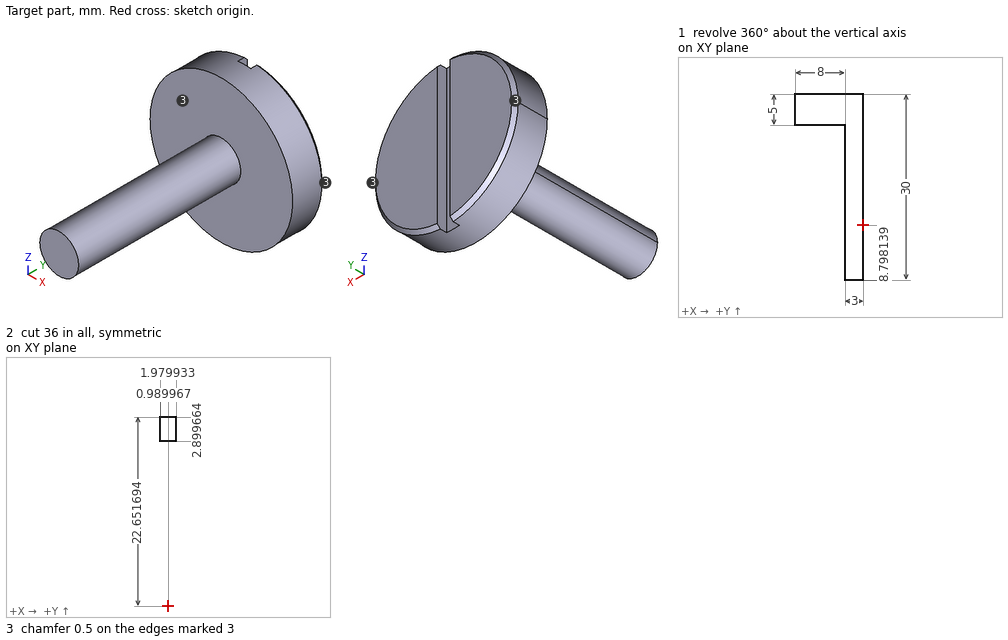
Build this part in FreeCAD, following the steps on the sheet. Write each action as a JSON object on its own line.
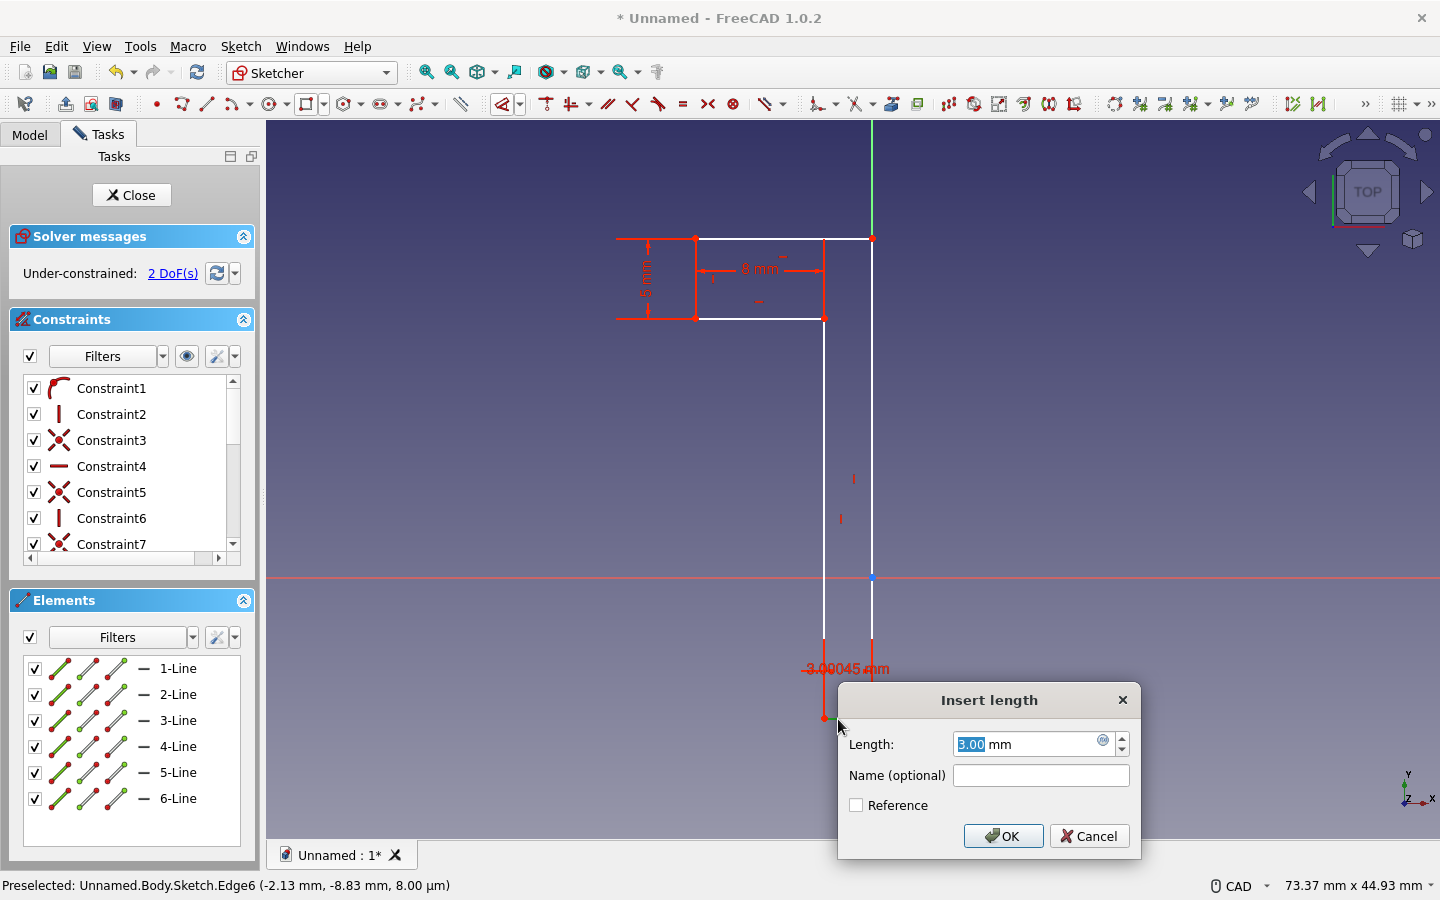
{"action": "type", "text": "3"}
{"action": "key", "text": "Return"}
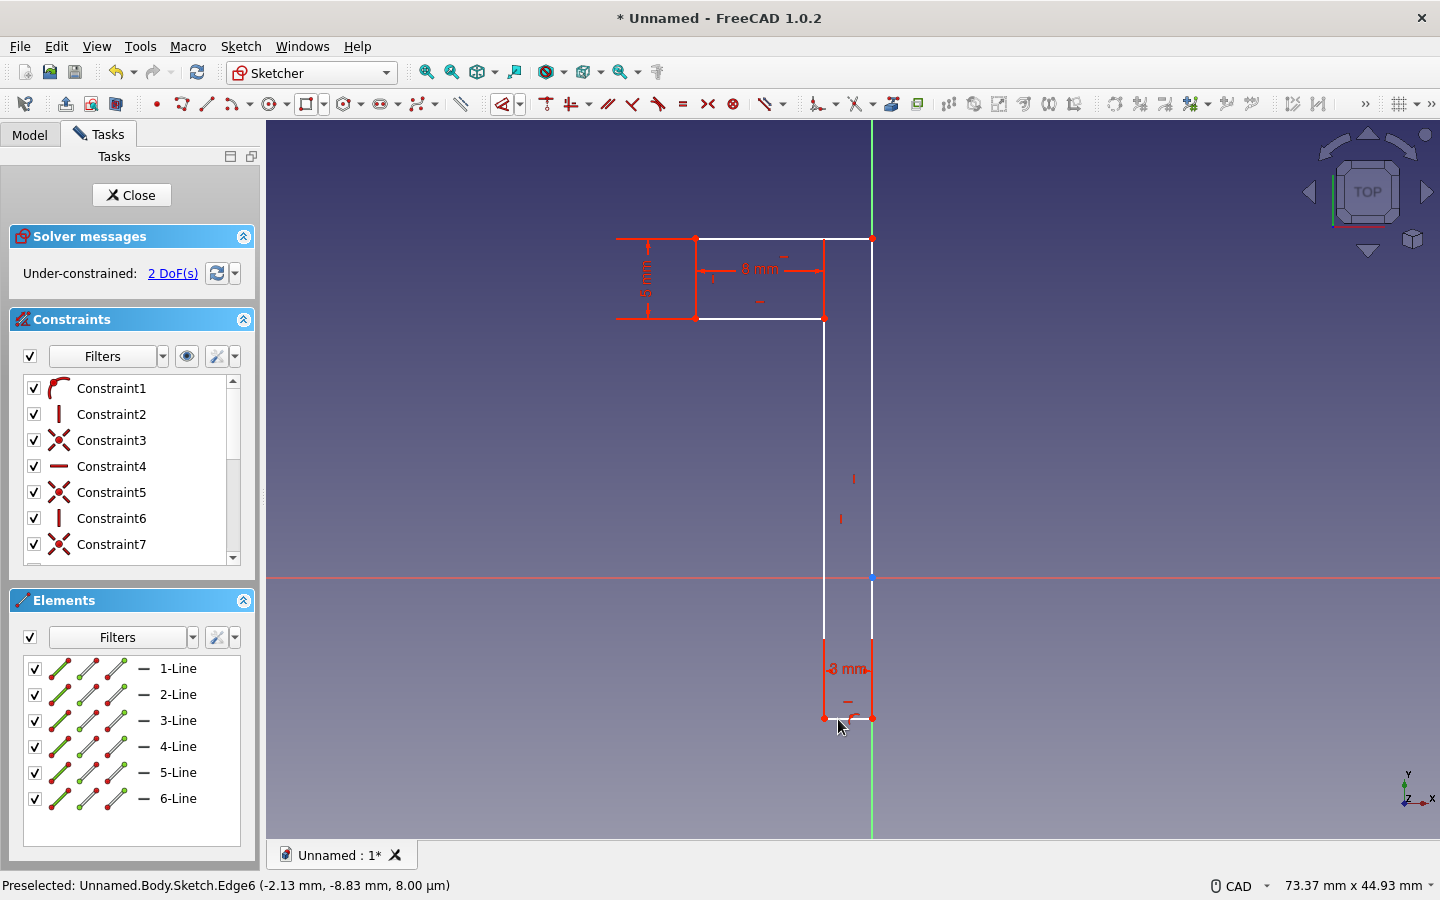
{"action": "left_click", "coordinate": [872, 383]}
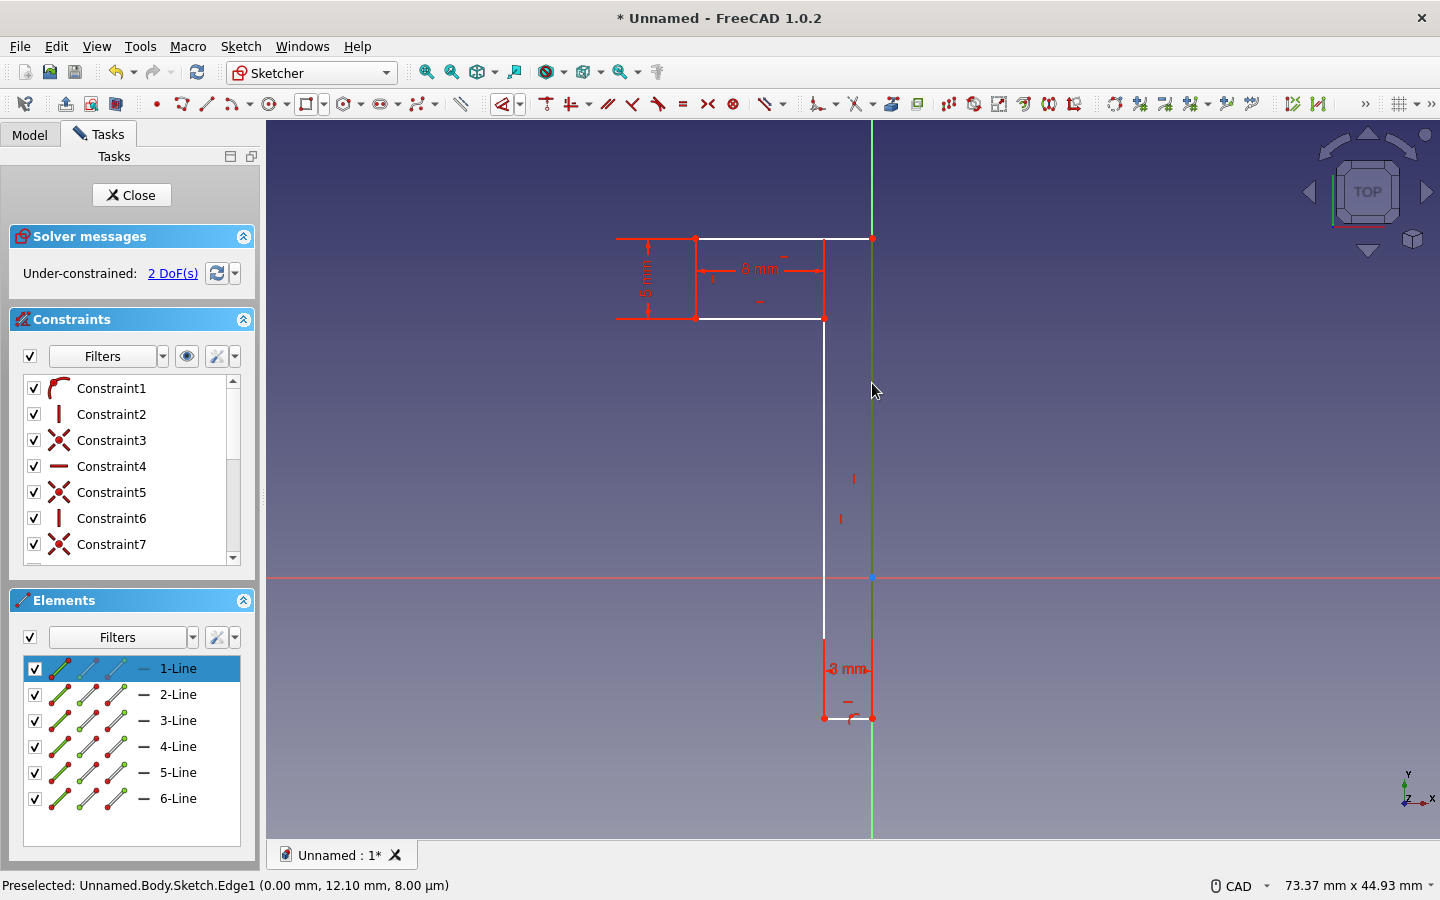
{"action": "left_click", "coordinate": [520, 104]}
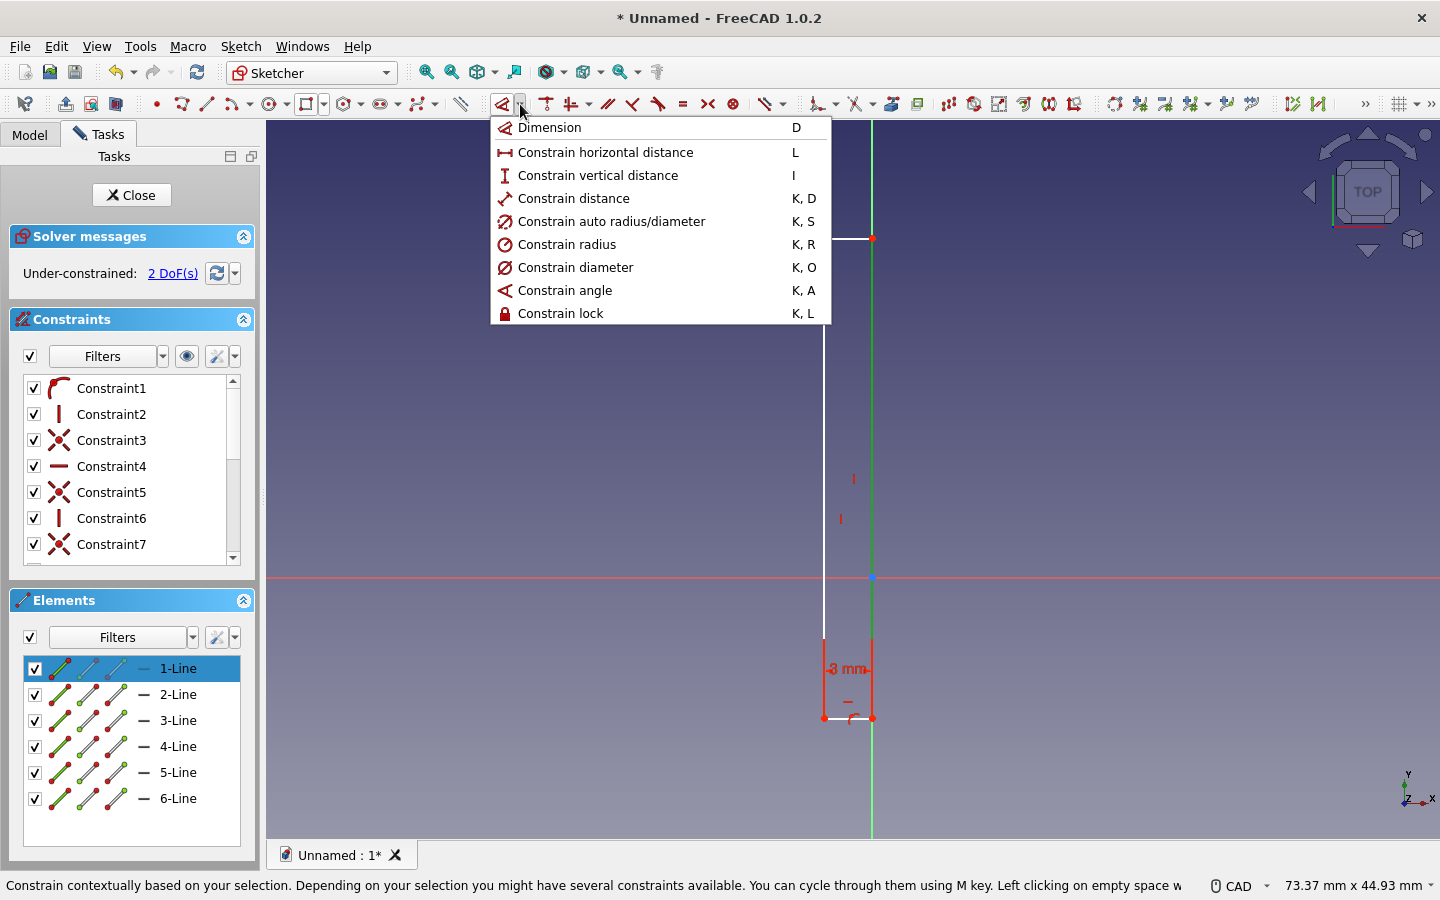
{"action": "left_click", "coordinate": [661, 176]}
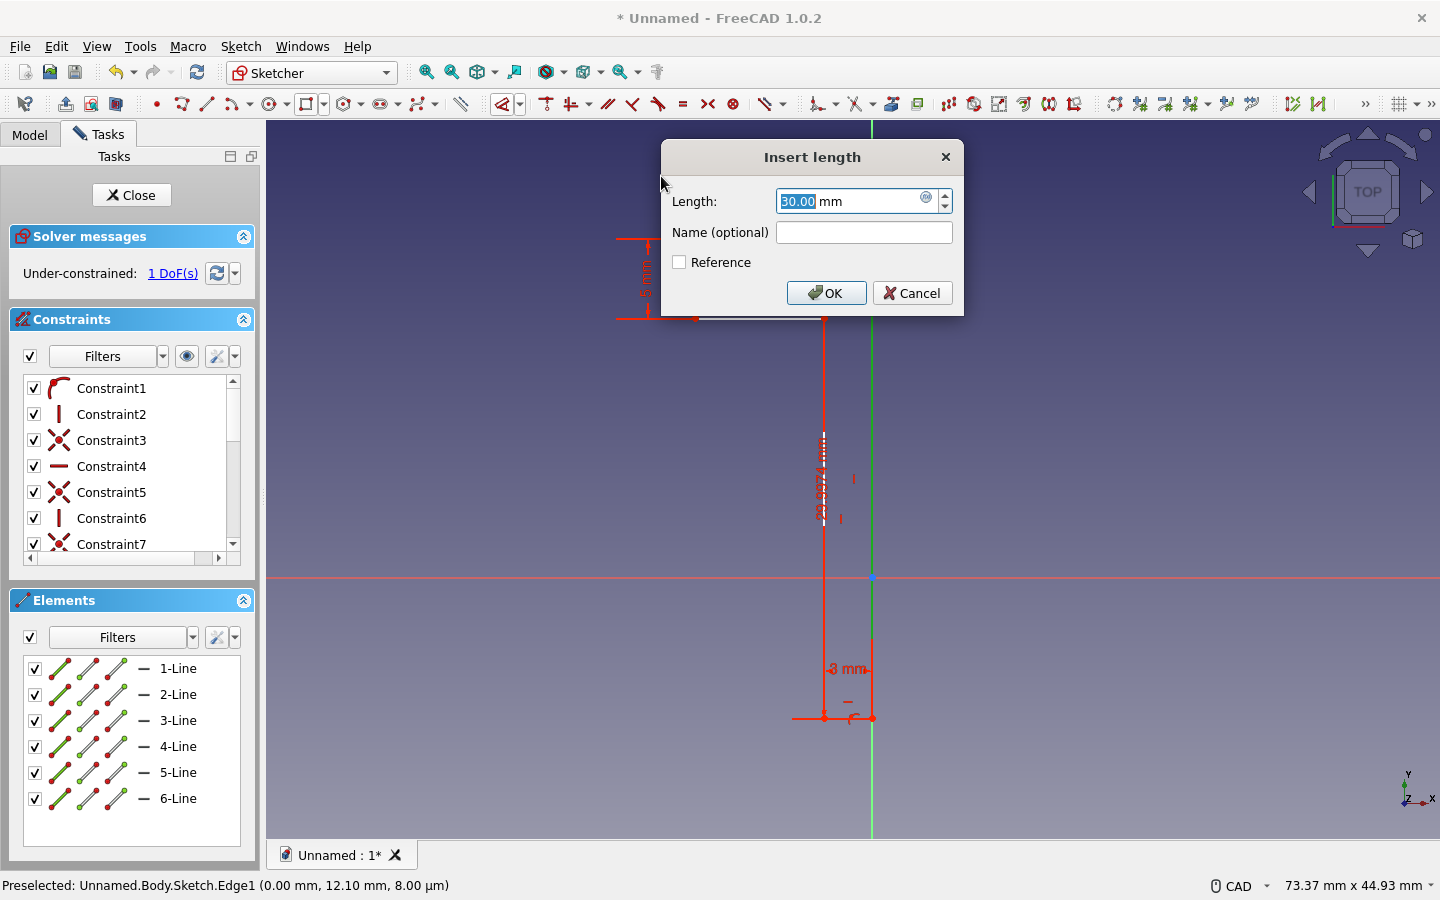
{"action": "type", "text": "30"}
{"action": "key", "text": "Return"}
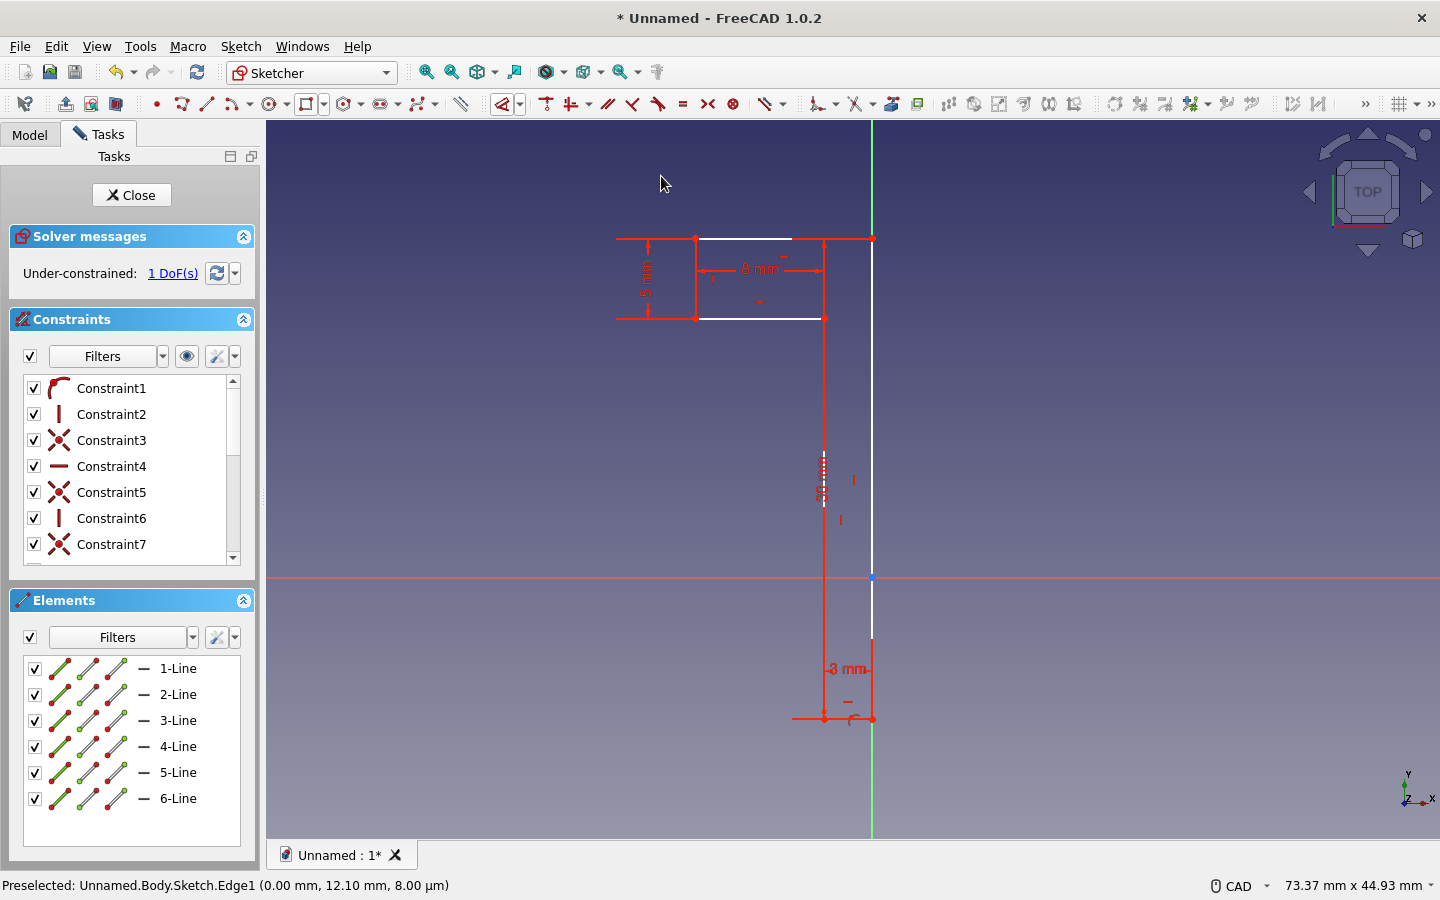
{"action": "left_click", "coordinate": [872, 719]}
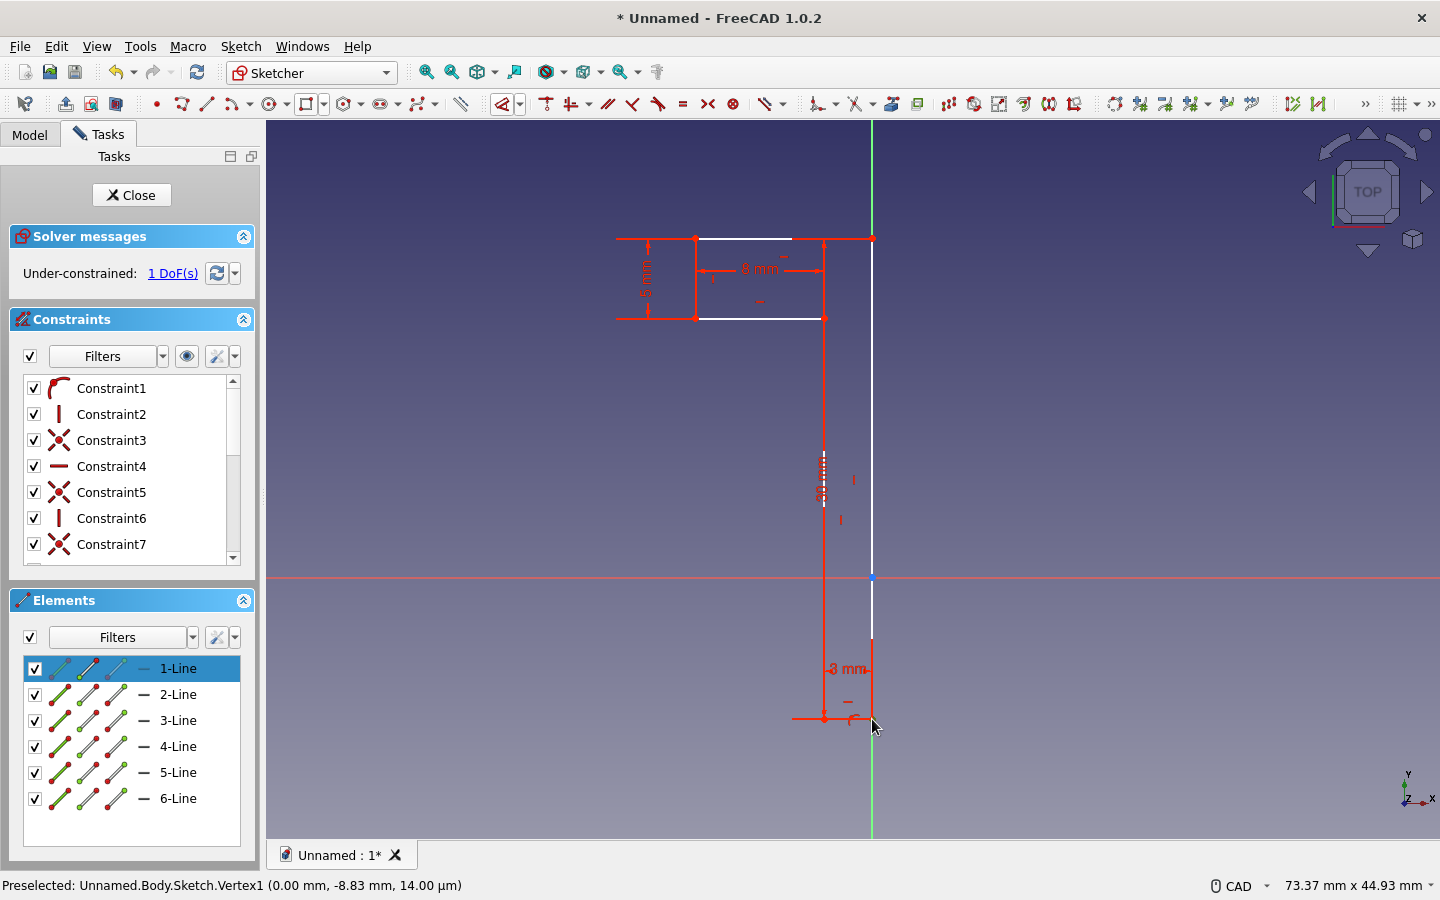
{"action": "key", "text": "i"}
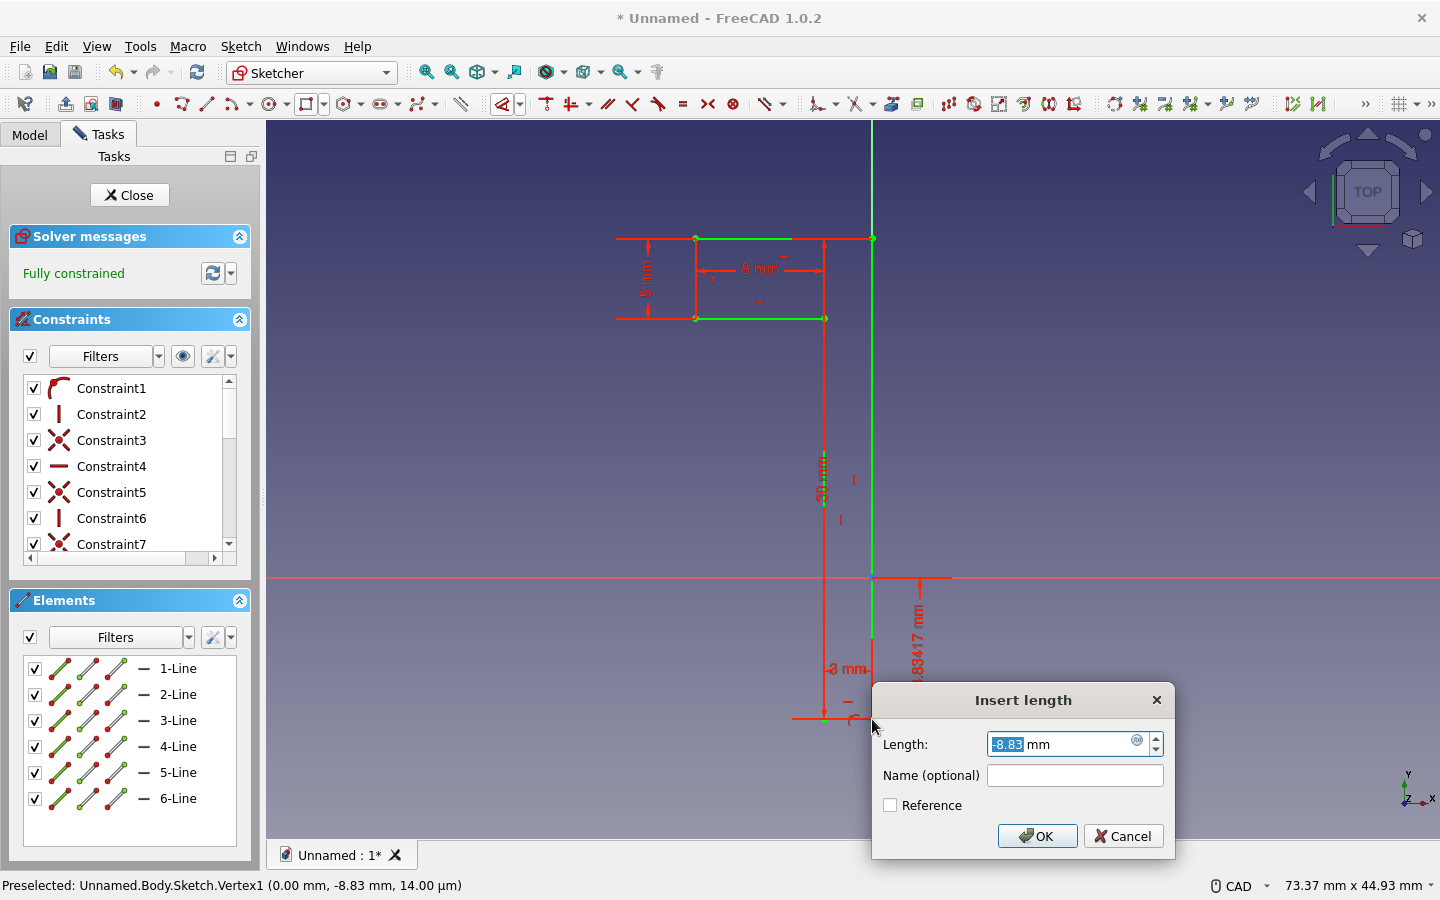
{"action": "type", "text": "-8.798139"}
{"action": "key", "text": "Return"}